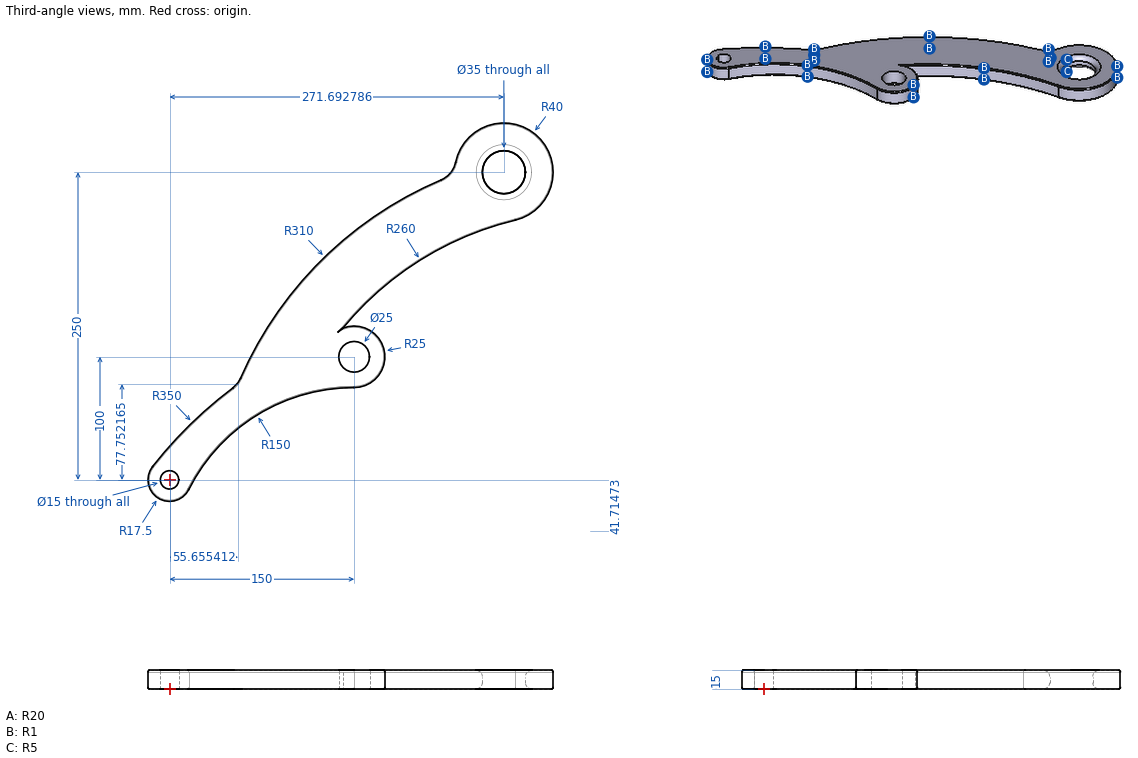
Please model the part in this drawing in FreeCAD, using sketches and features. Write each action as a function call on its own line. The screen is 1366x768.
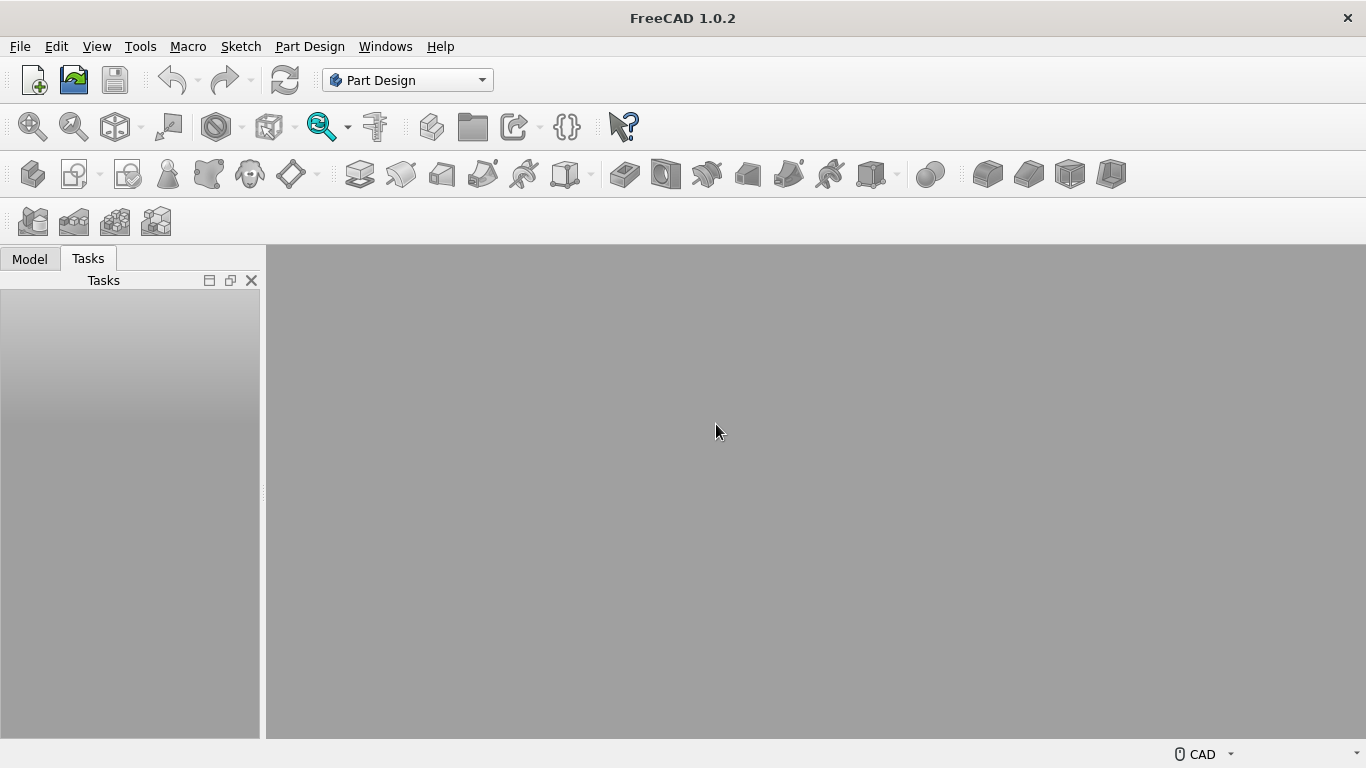
click(33, 80)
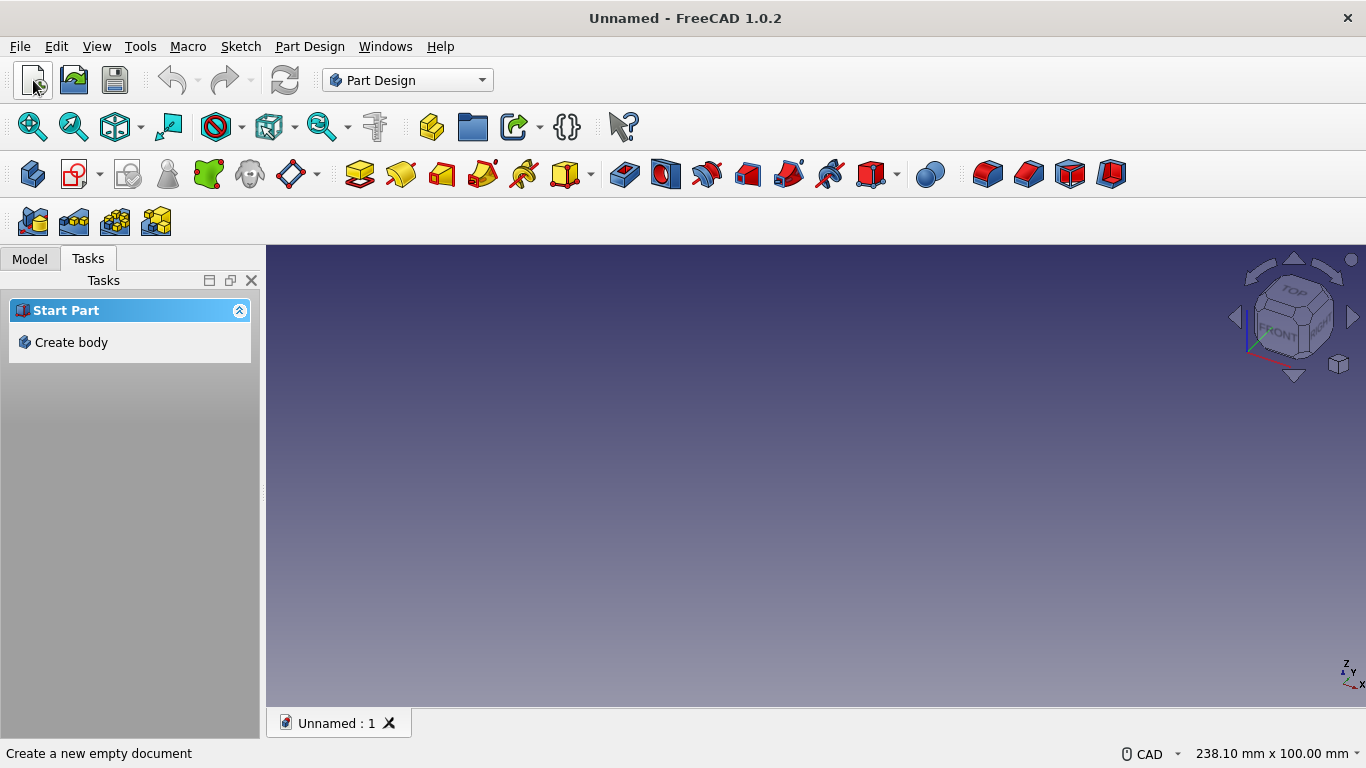
click(33, 174)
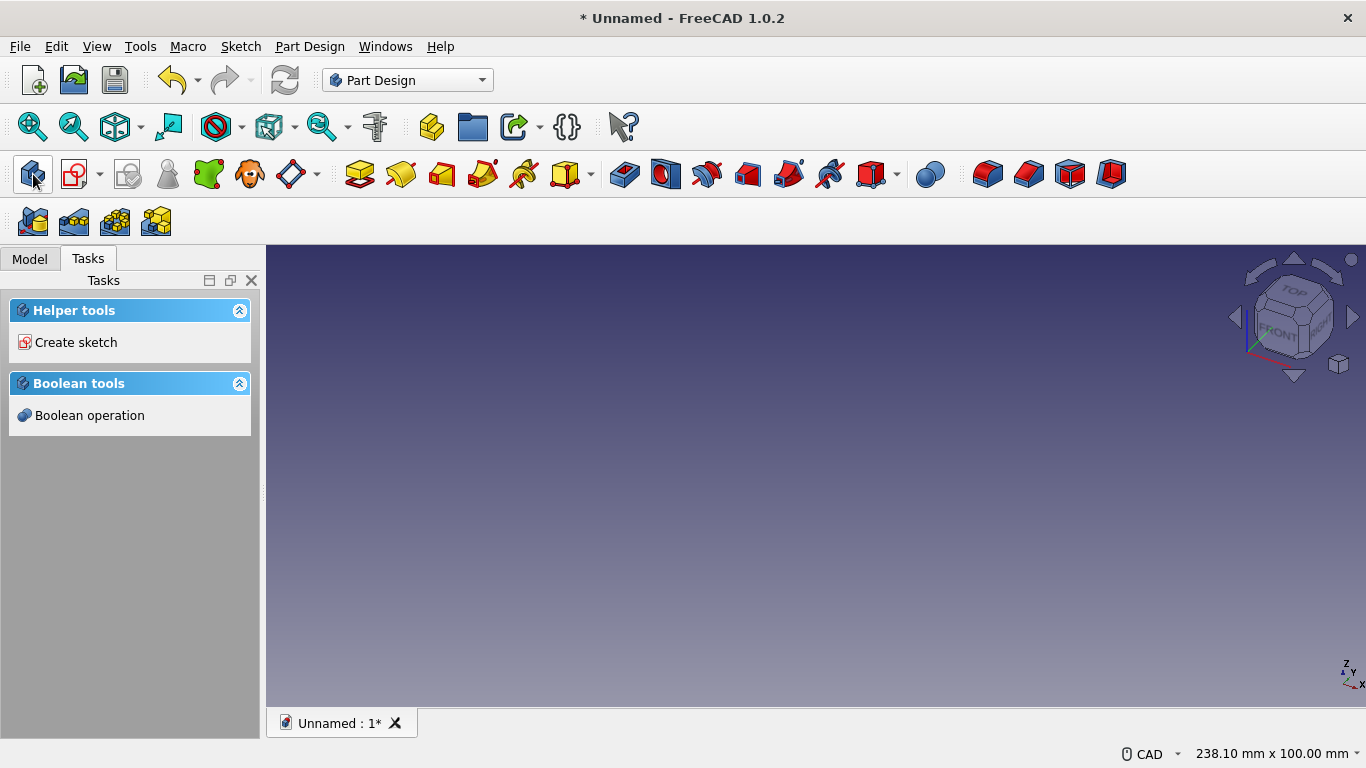
click(30, 258)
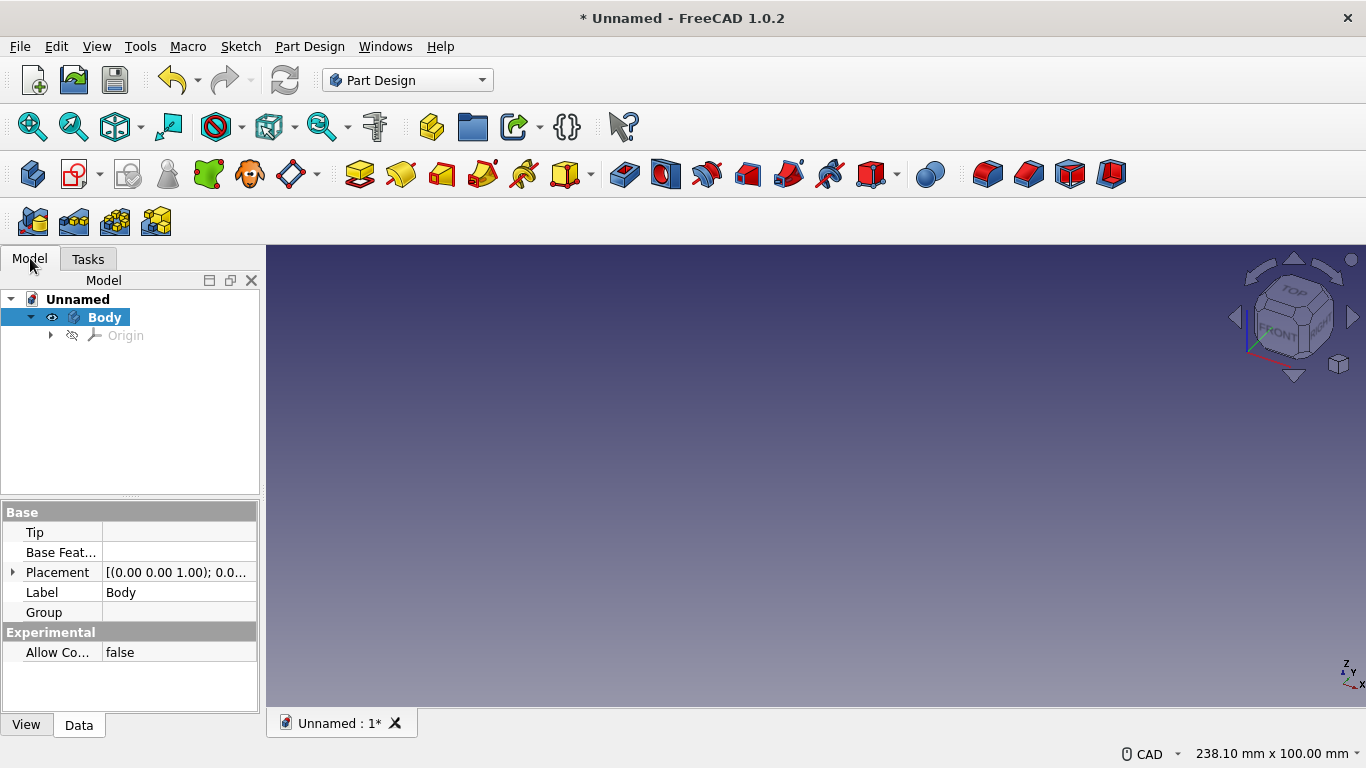
click(51, 335)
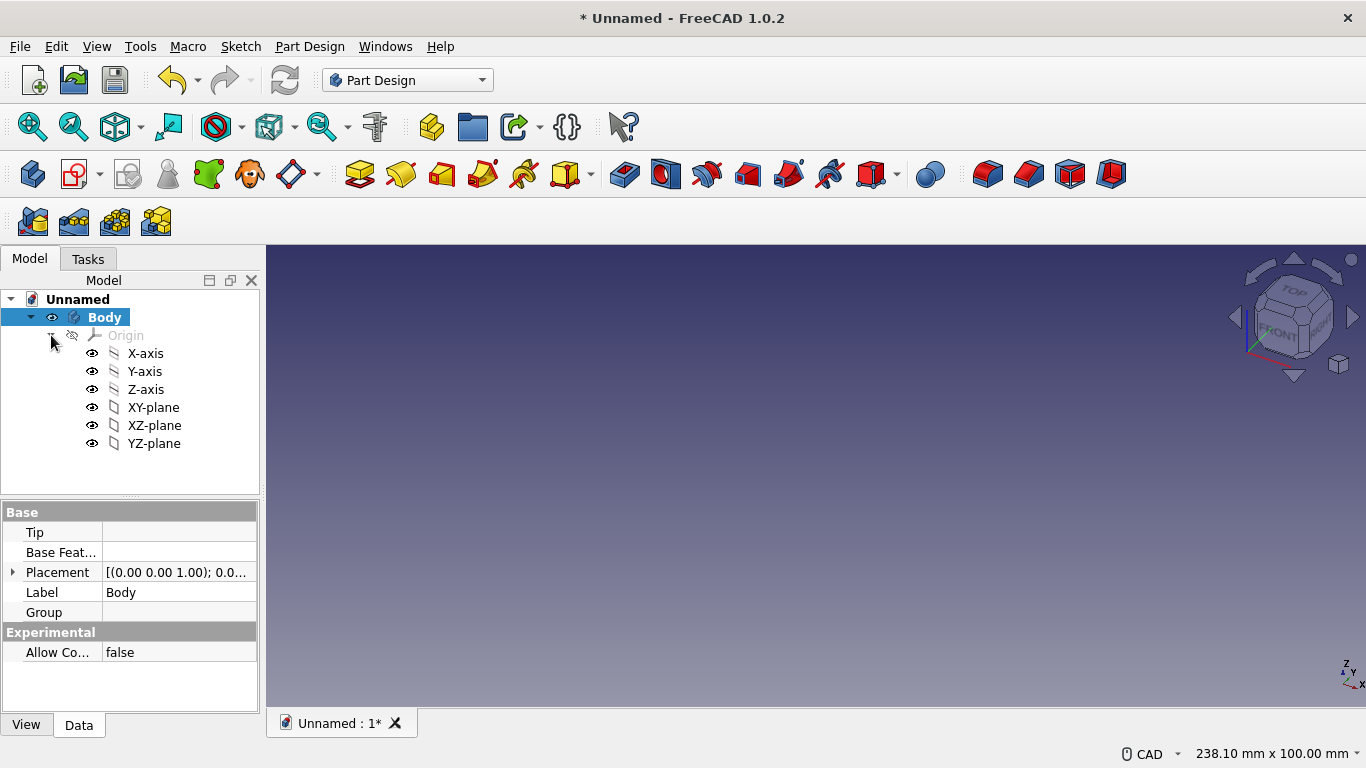
click(137, 407)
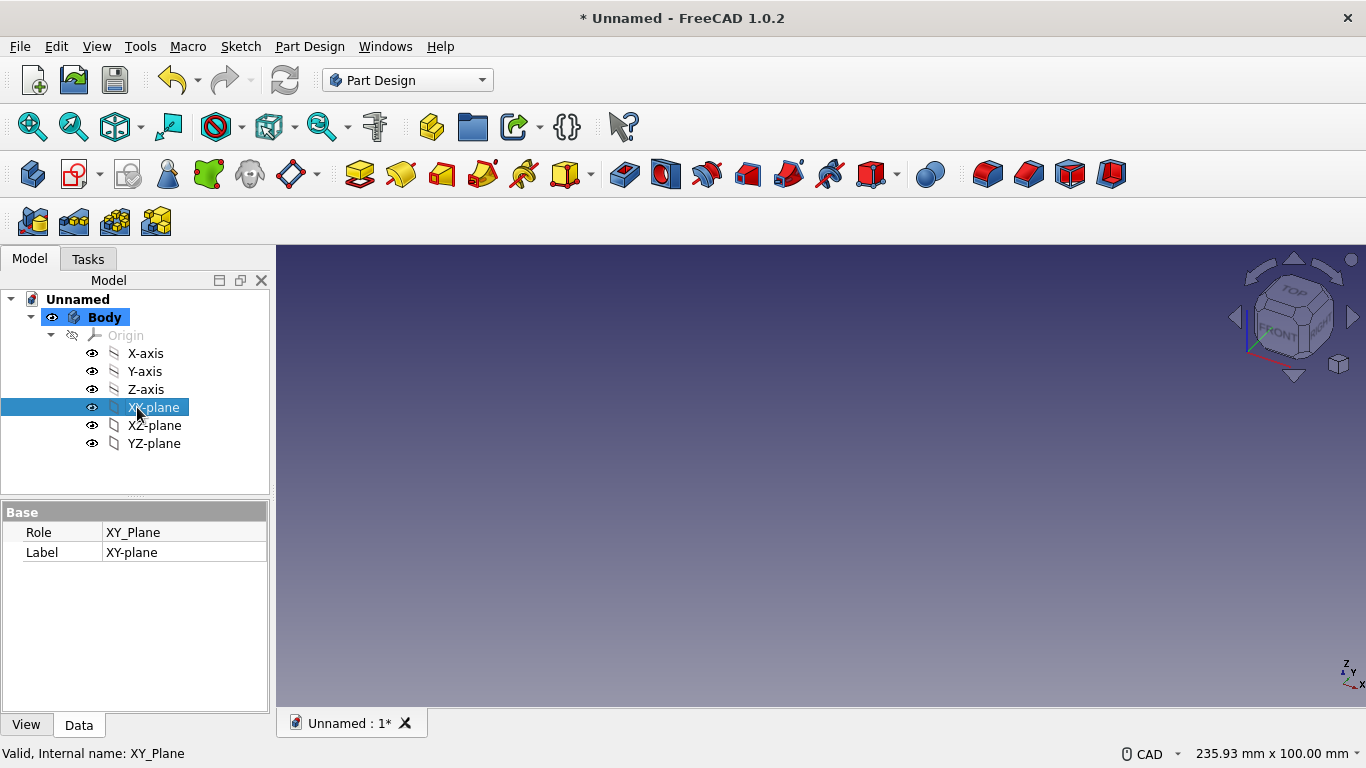
click(290, 174)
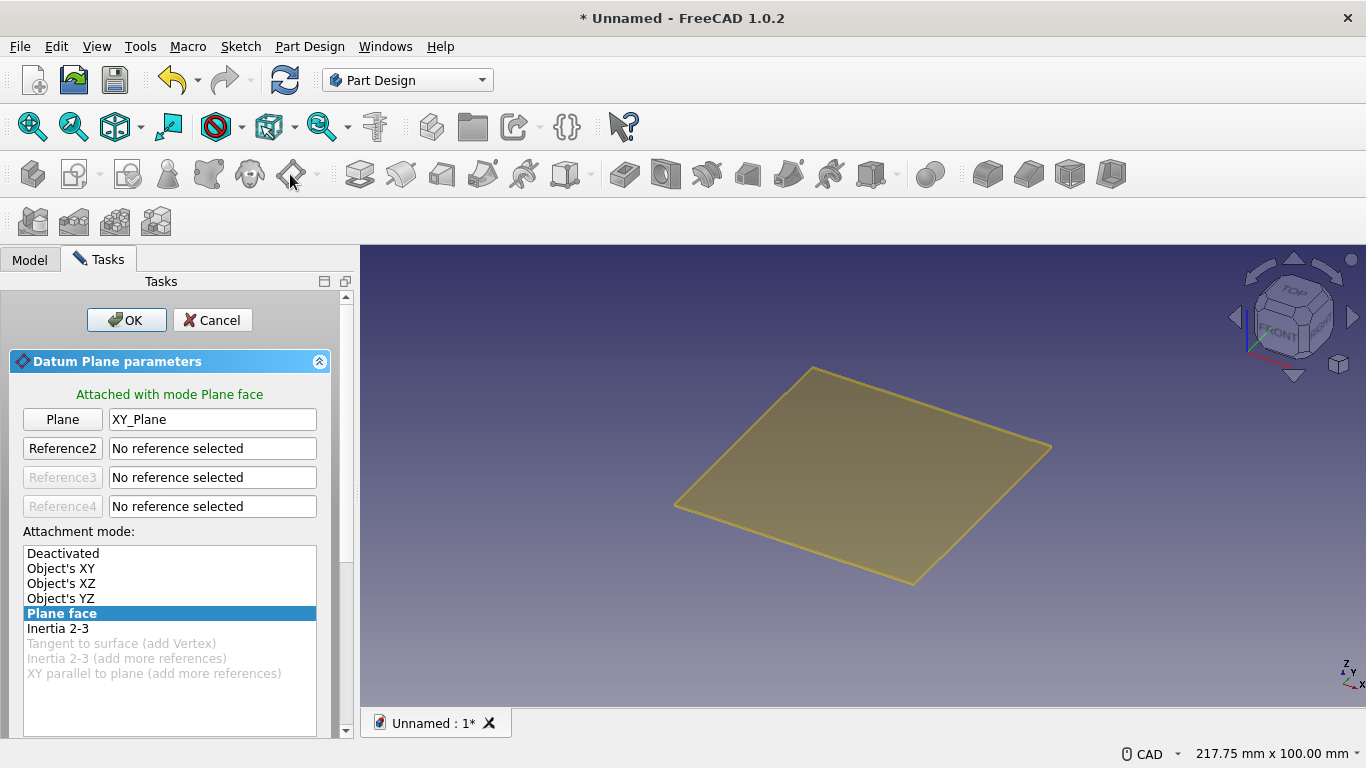
scroll(346, 514, down, 4)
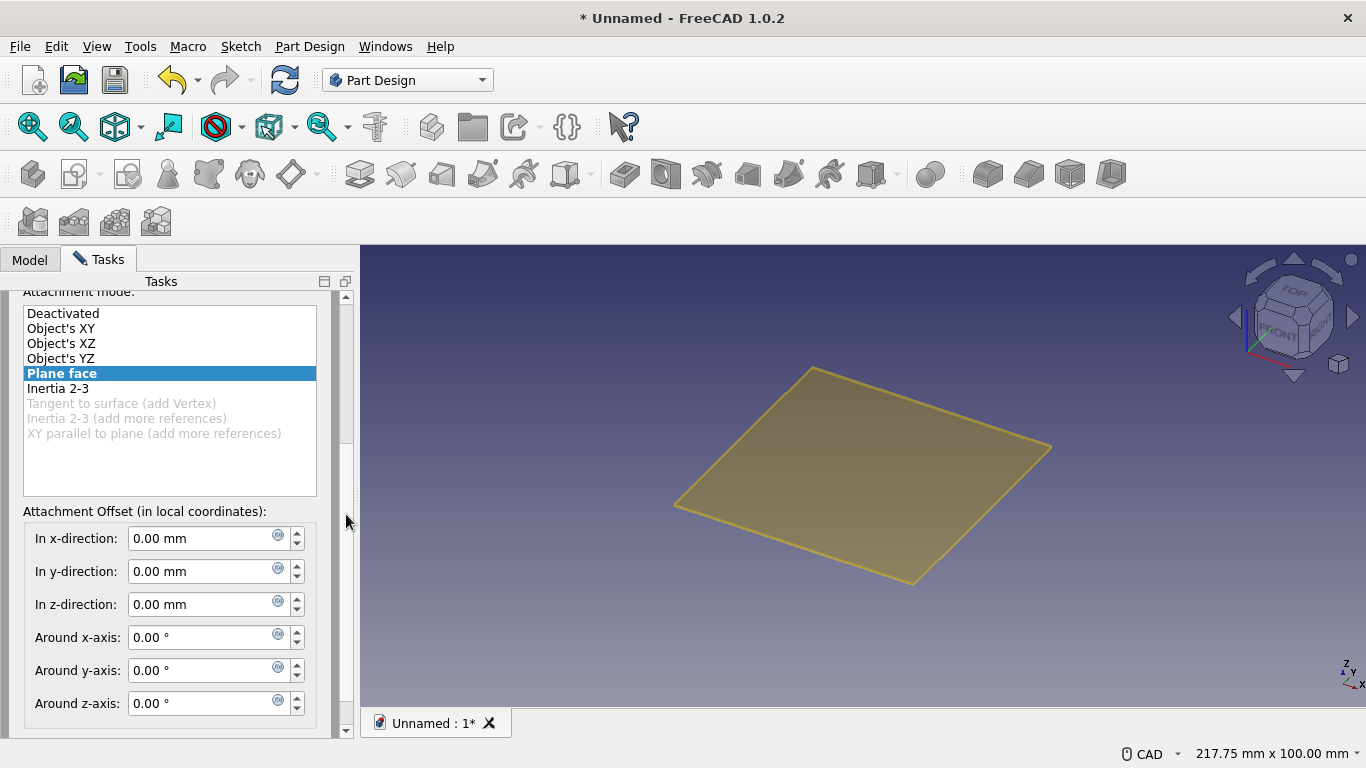
triple_click(210, 604)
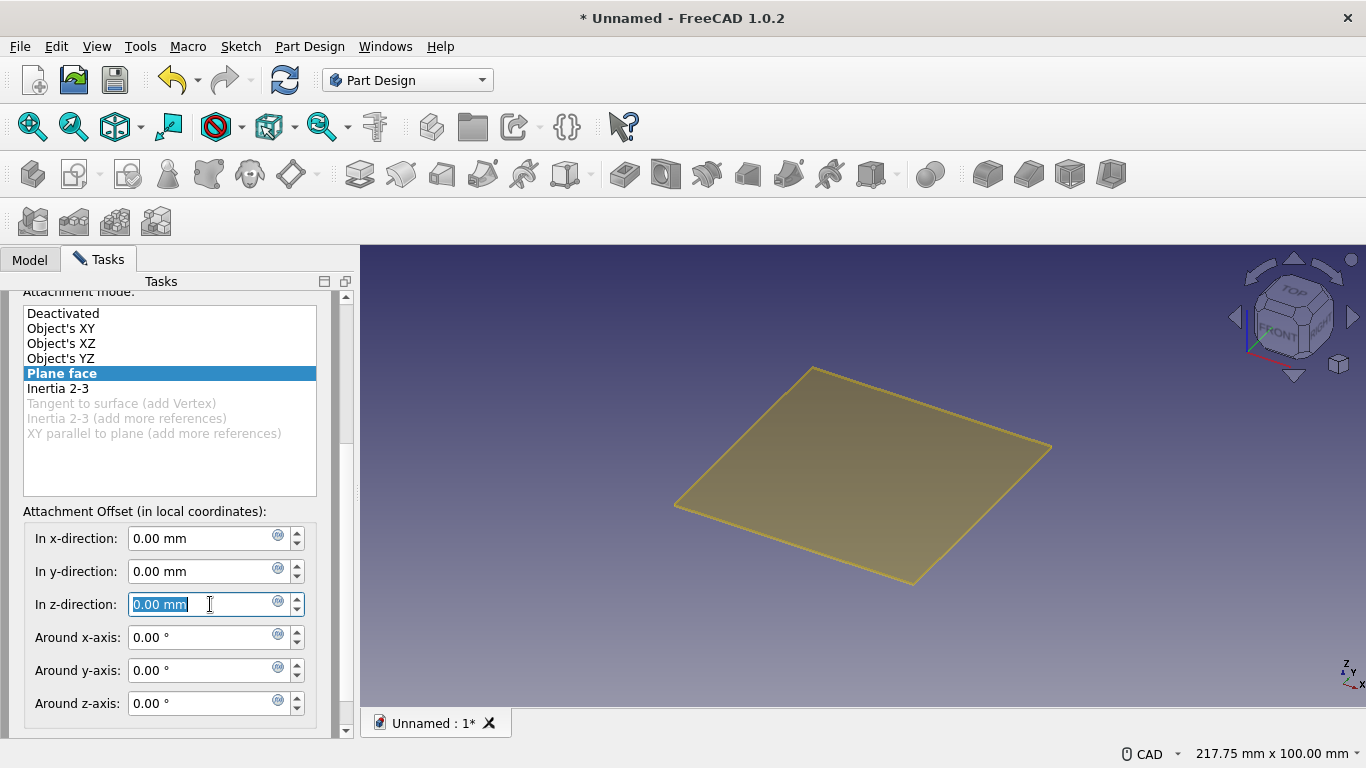
text(15)
key(Tab)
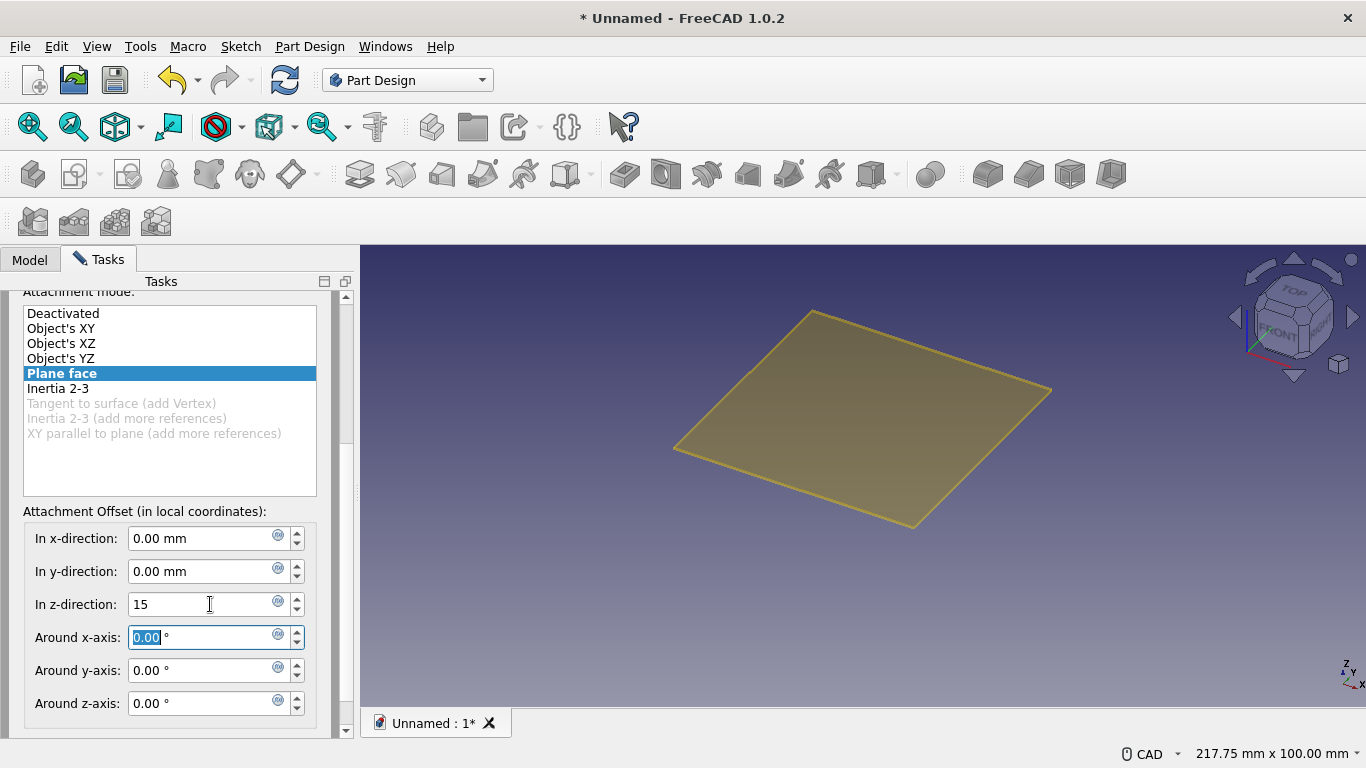
scroll(346, 514, up, 5)